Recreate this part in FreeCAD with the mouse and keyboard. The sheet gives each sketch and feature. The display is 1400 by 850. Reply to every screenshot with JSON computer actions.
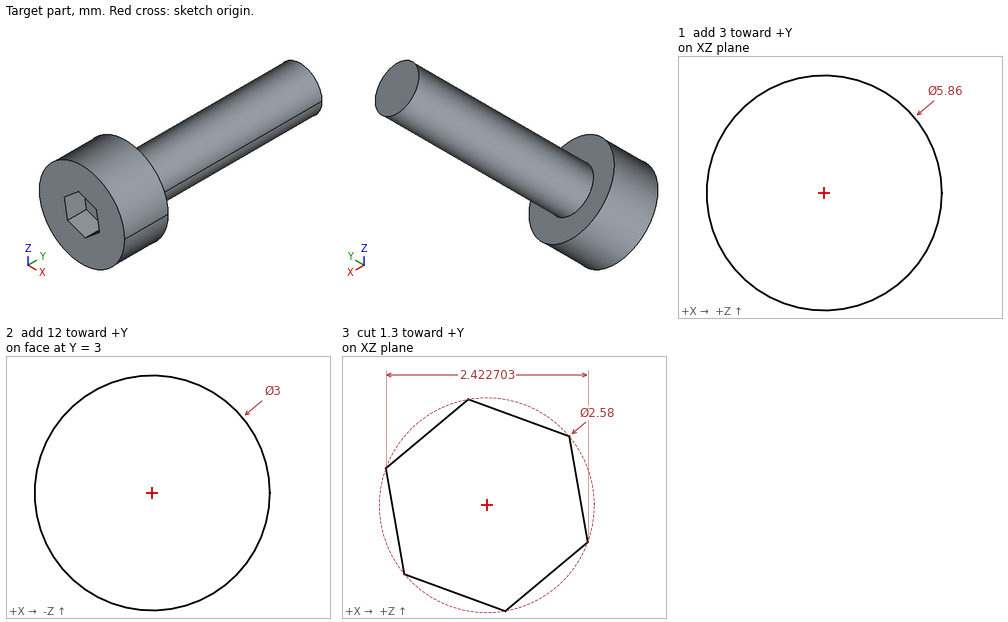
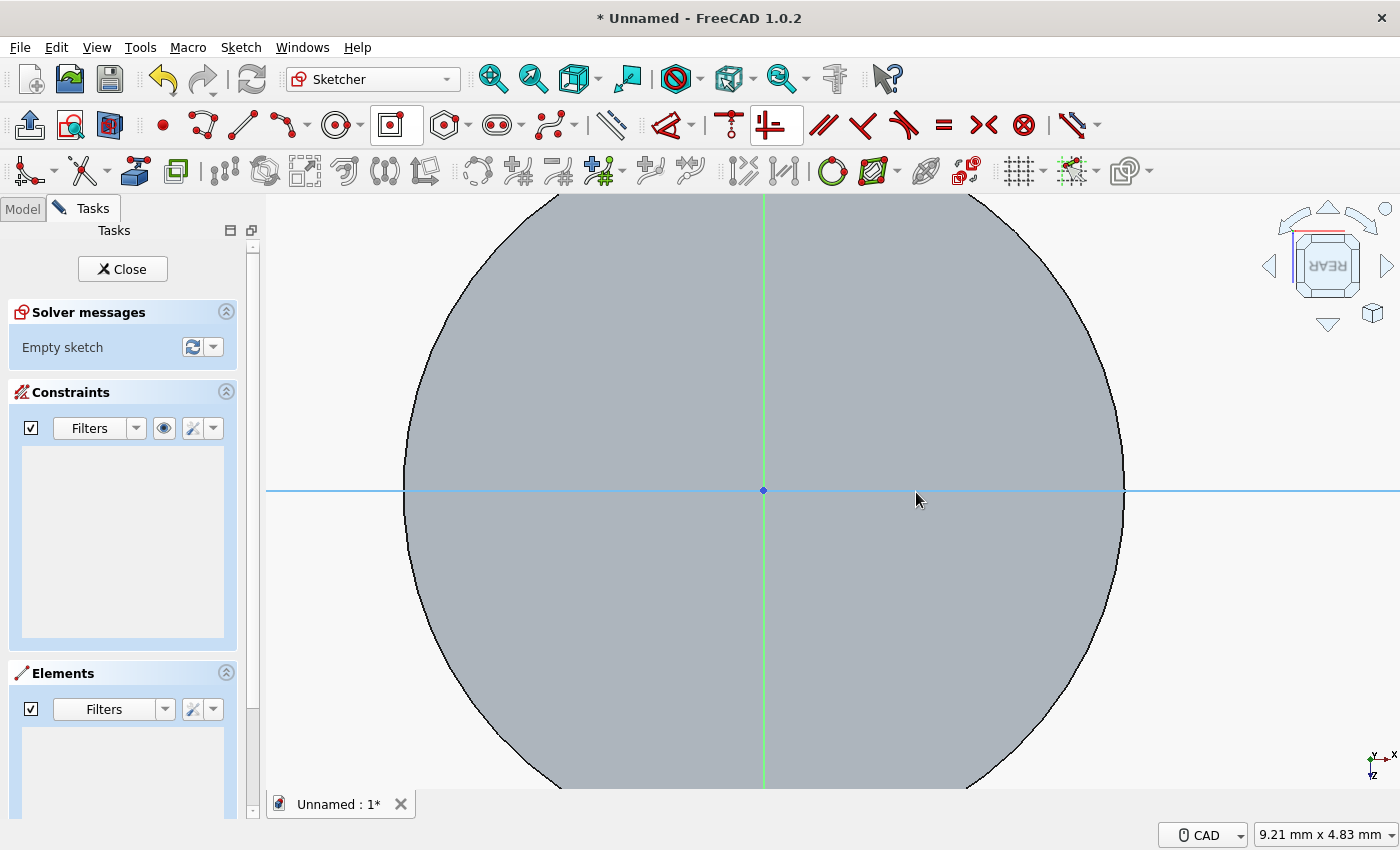
{"action": "left_click", "coordinate": [336, 126]}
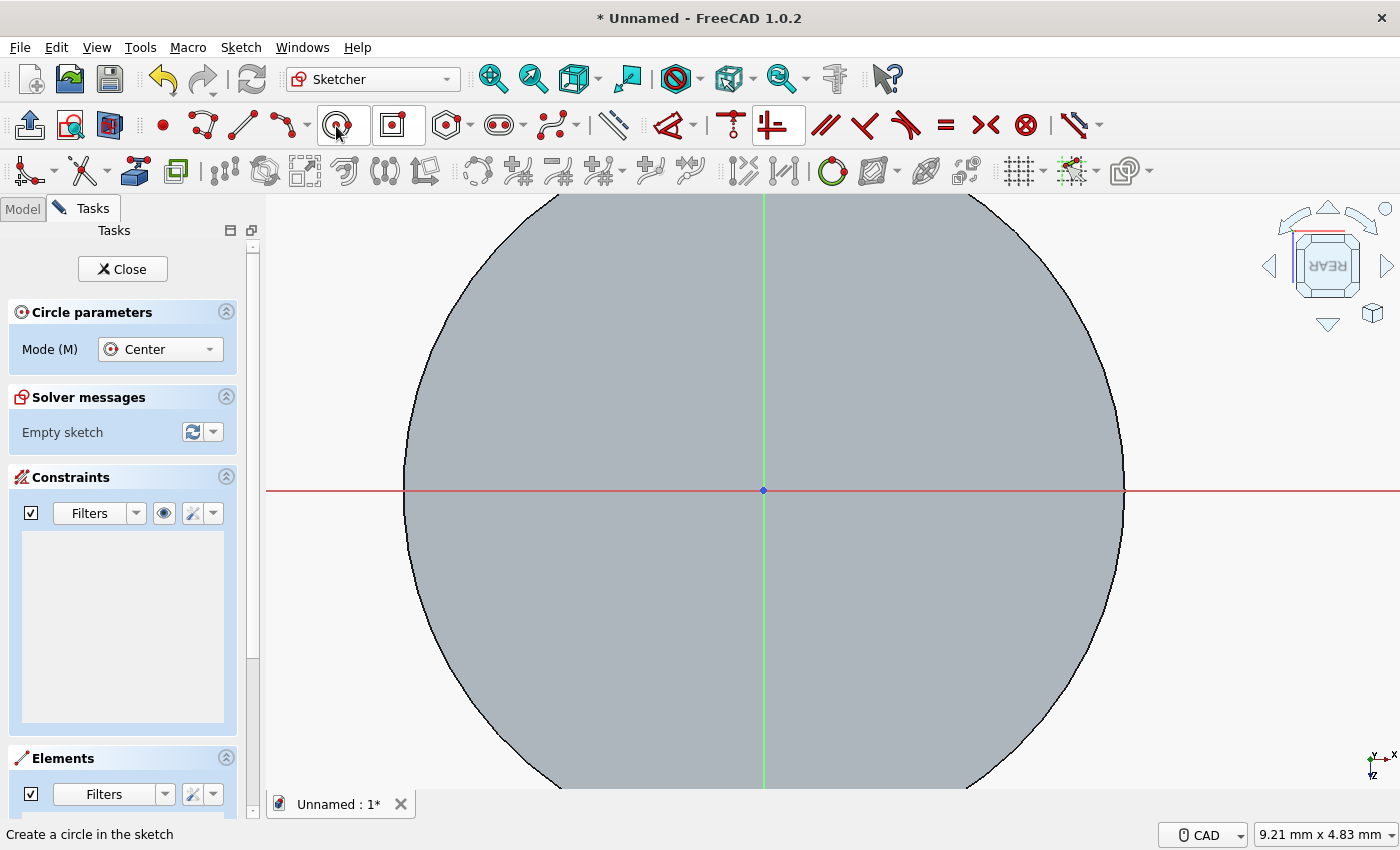
{"action": "left_click", "coordinate": [764, 491]}
{"action": "mouse_move", "coordinate": [895, 360]}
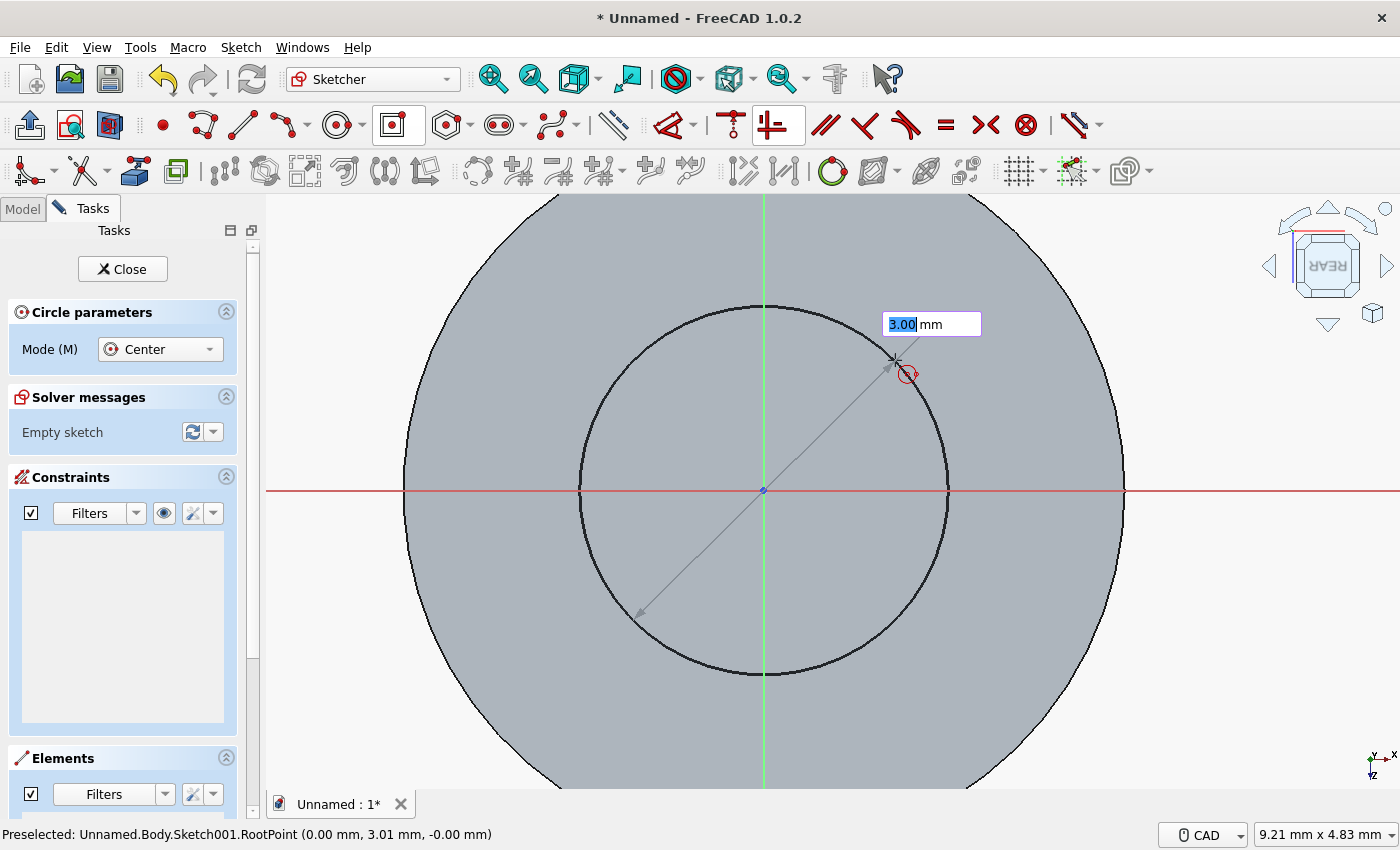
{"action": "type", "text": "3"}
{"action": "key", "text": "Return"}
{"action": "key", "text": "Escape"}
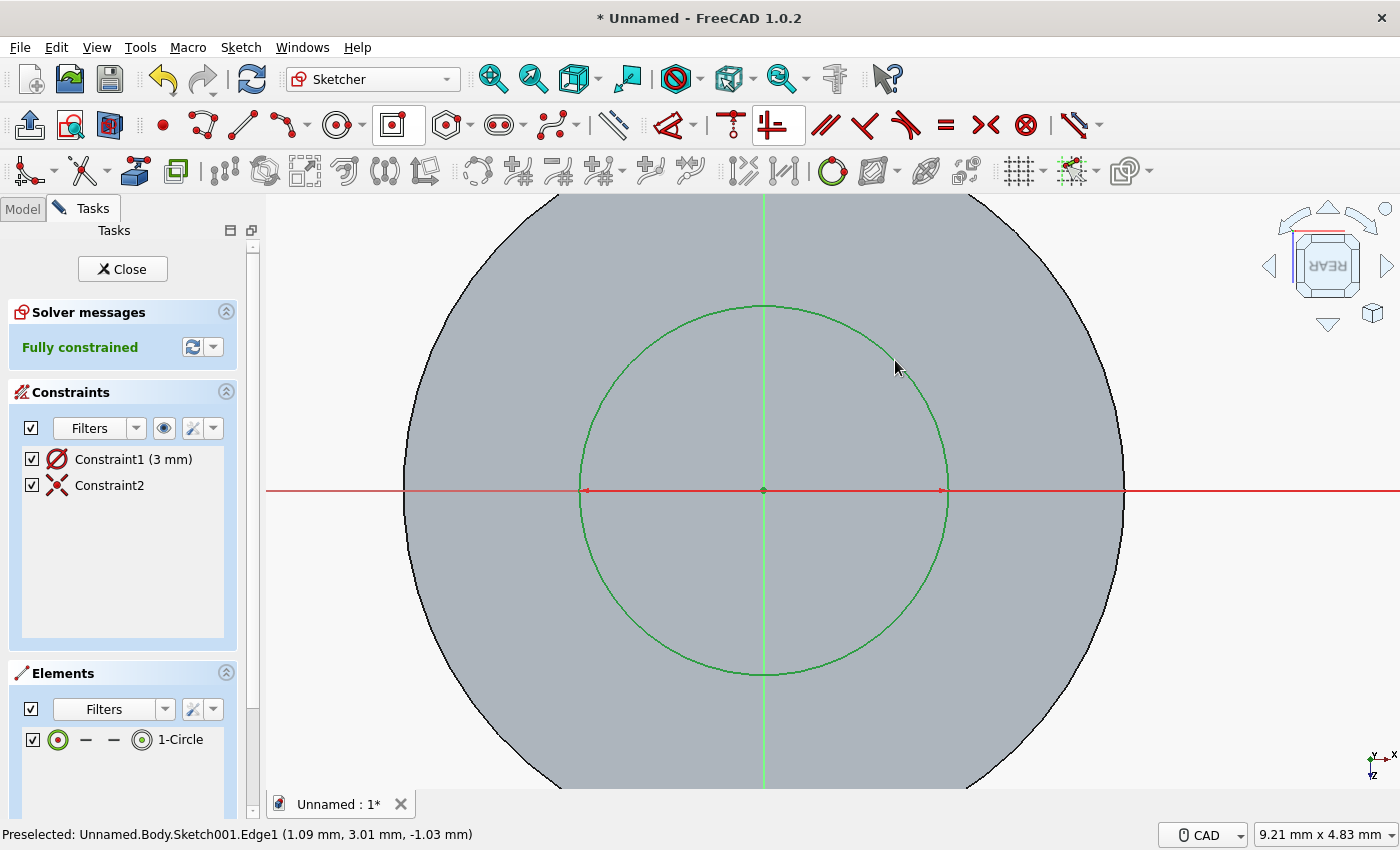
{"action": "left_click", "coordinate": [123, 269]}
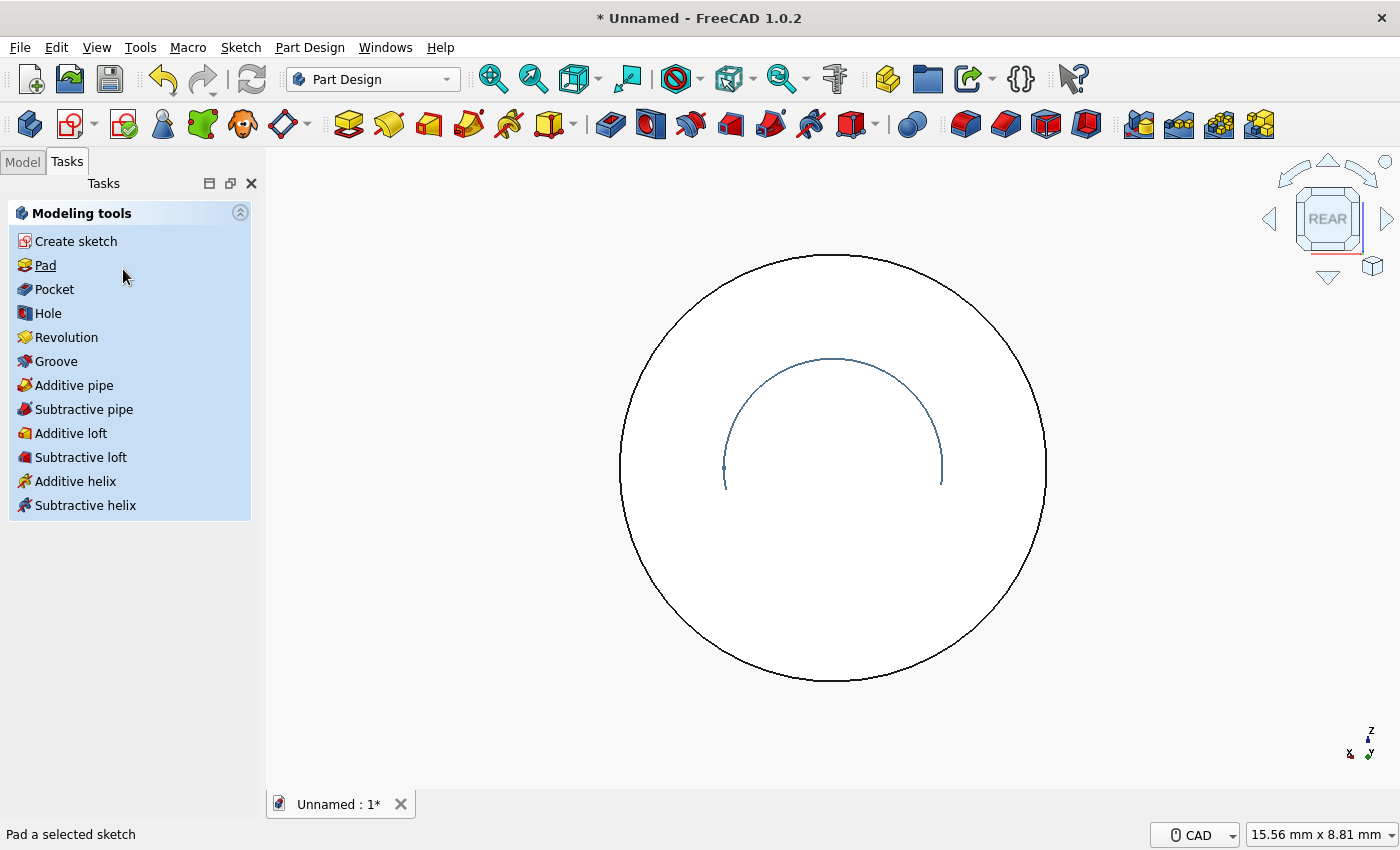
{"action": "left_click", "coordinate": [350, 124]}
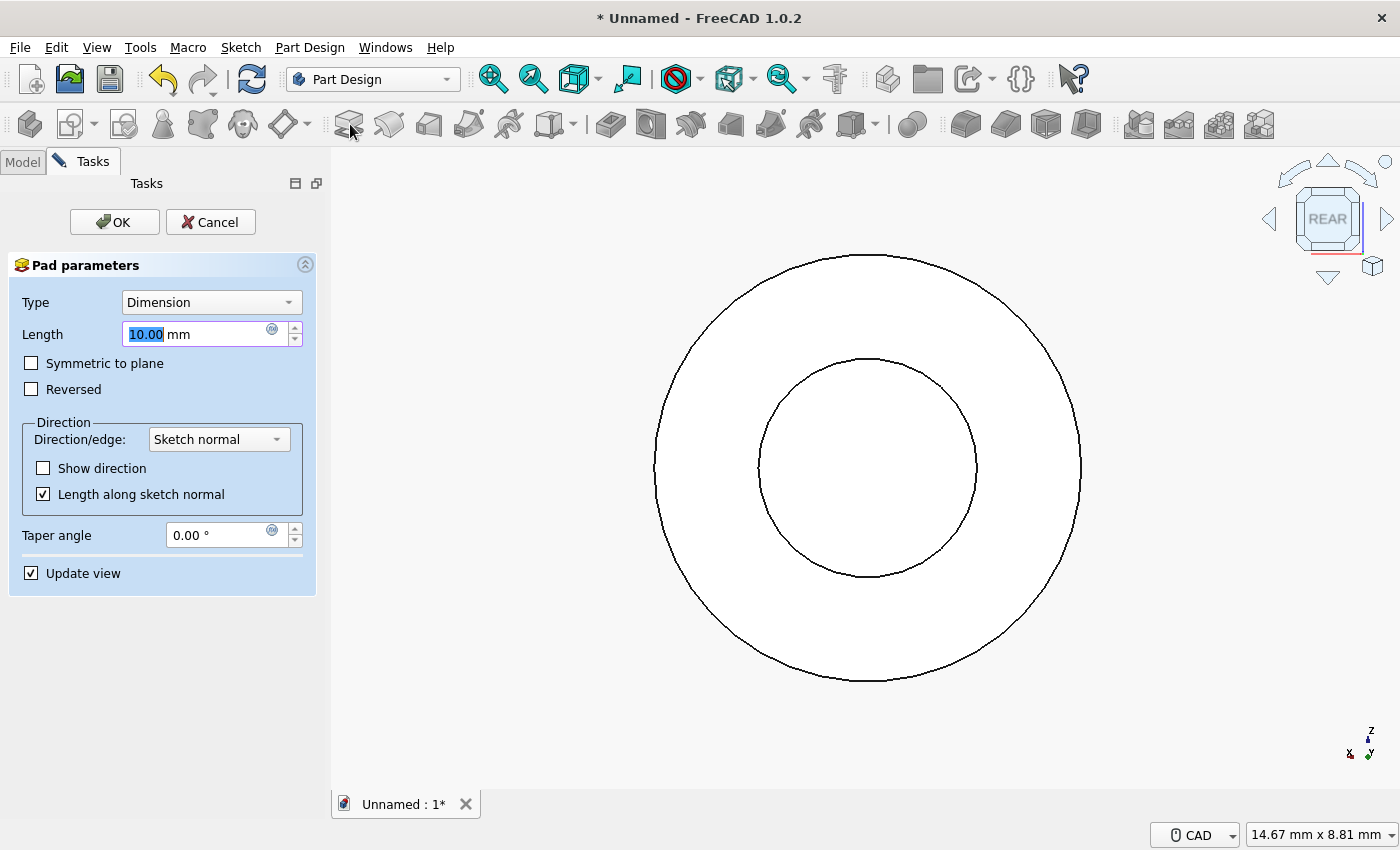
{"action": "type", "text": "12"}
{"action": "key", "text": "Tab"}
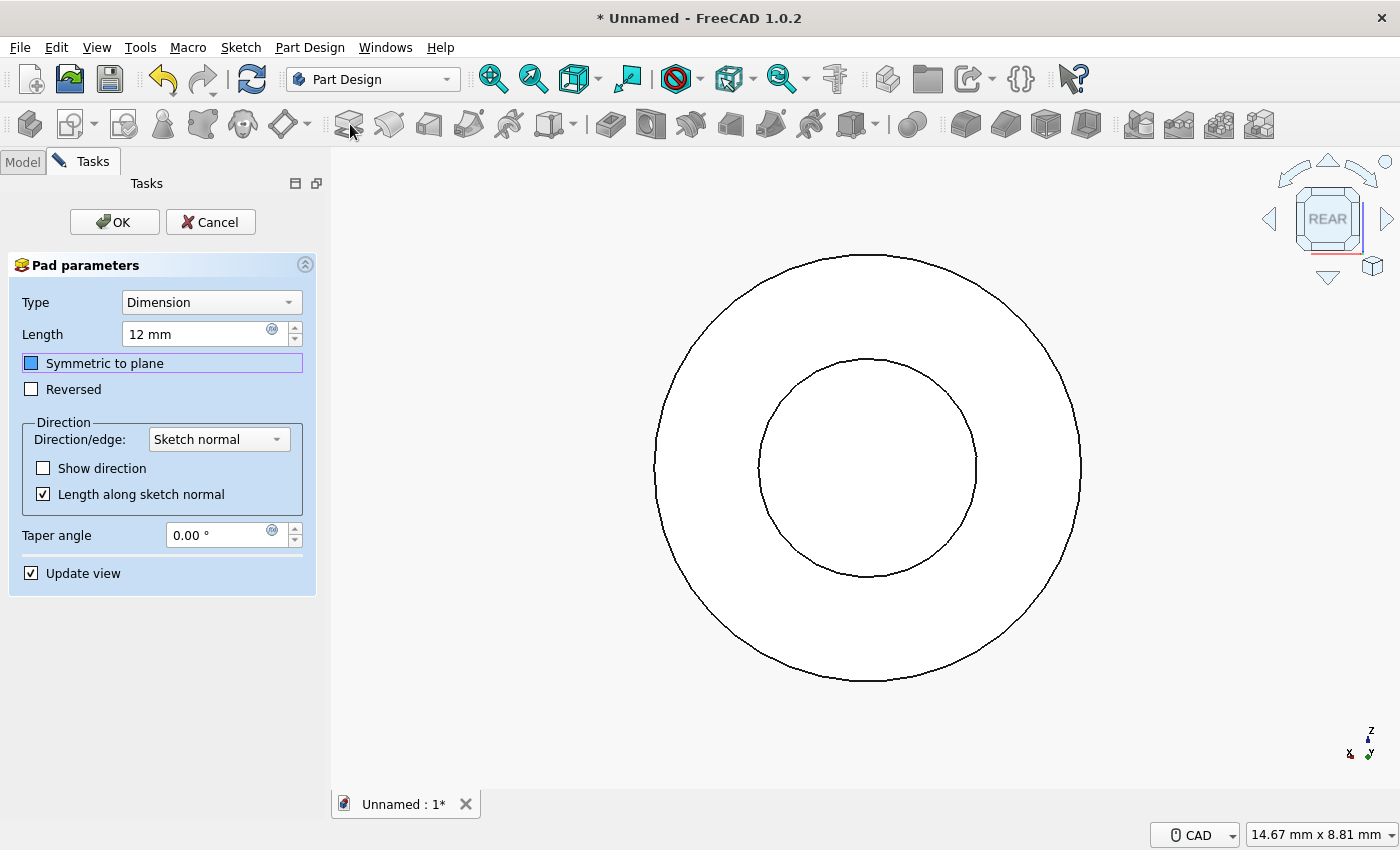
{"action": "left_click", "coordinate": [115, 222]}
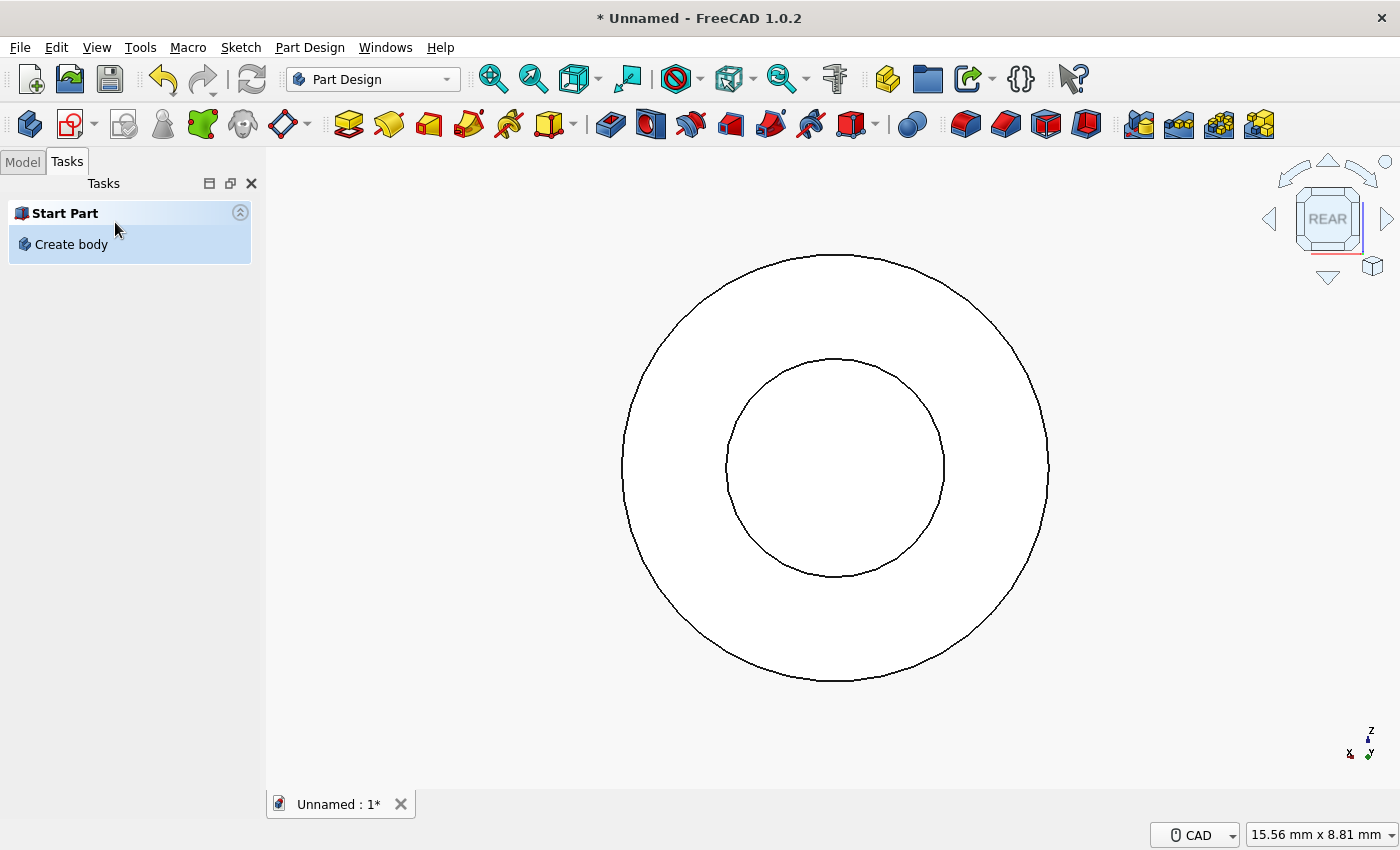
{"action": "left_click", "coordinate": [70, 124]}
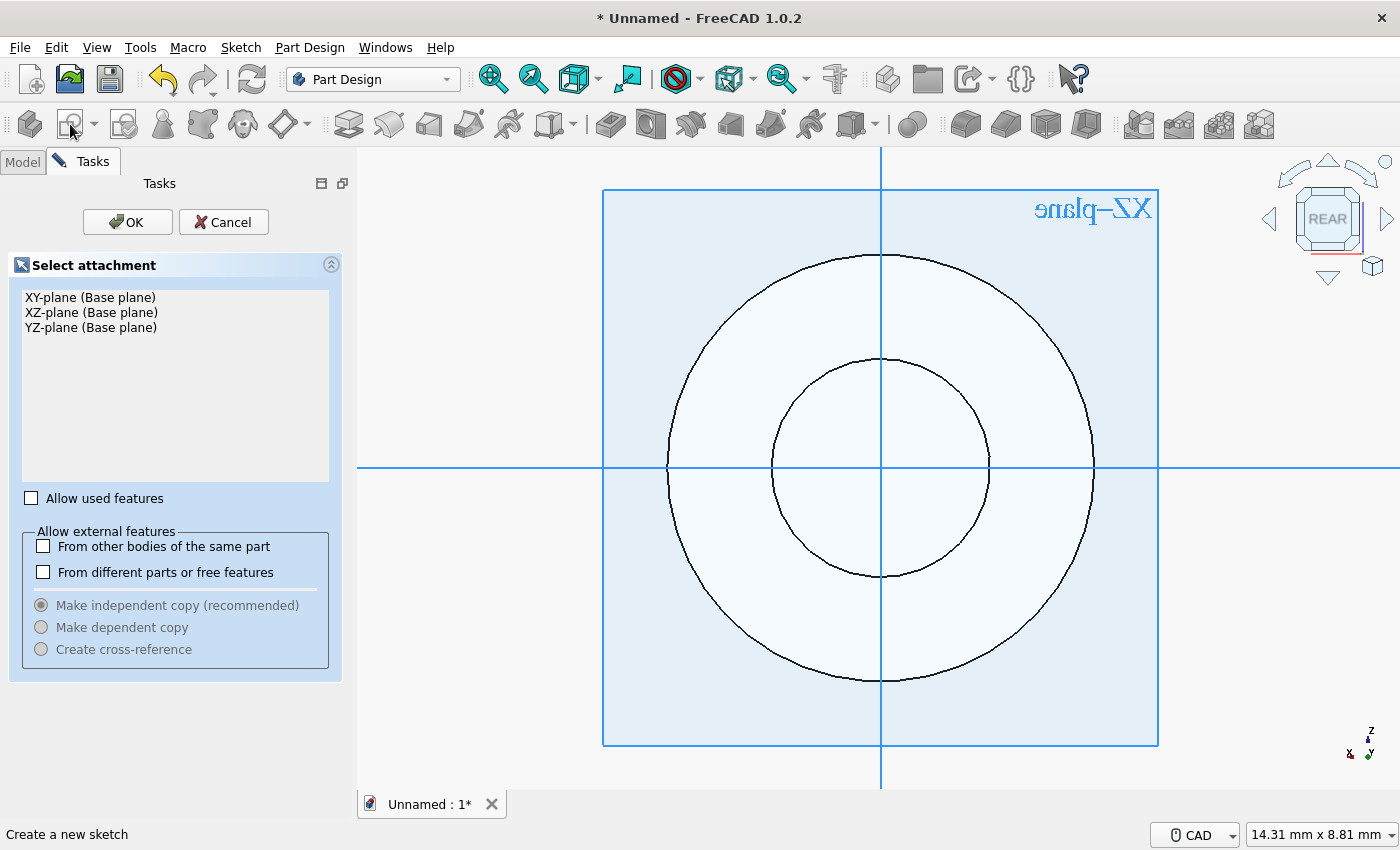
{"action": "left_click", "coordinate": [82, 312]}